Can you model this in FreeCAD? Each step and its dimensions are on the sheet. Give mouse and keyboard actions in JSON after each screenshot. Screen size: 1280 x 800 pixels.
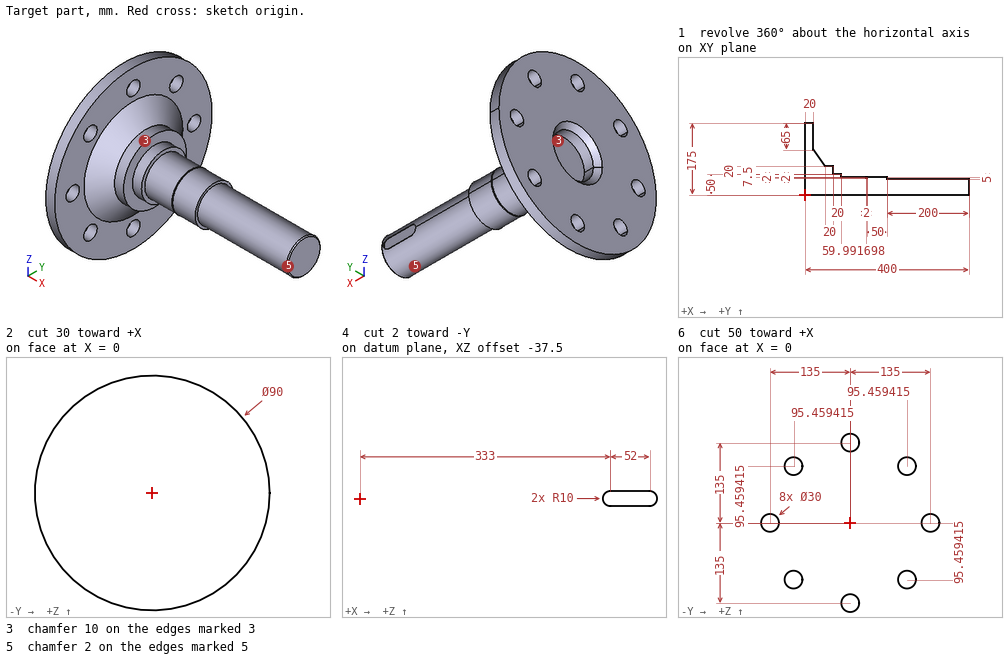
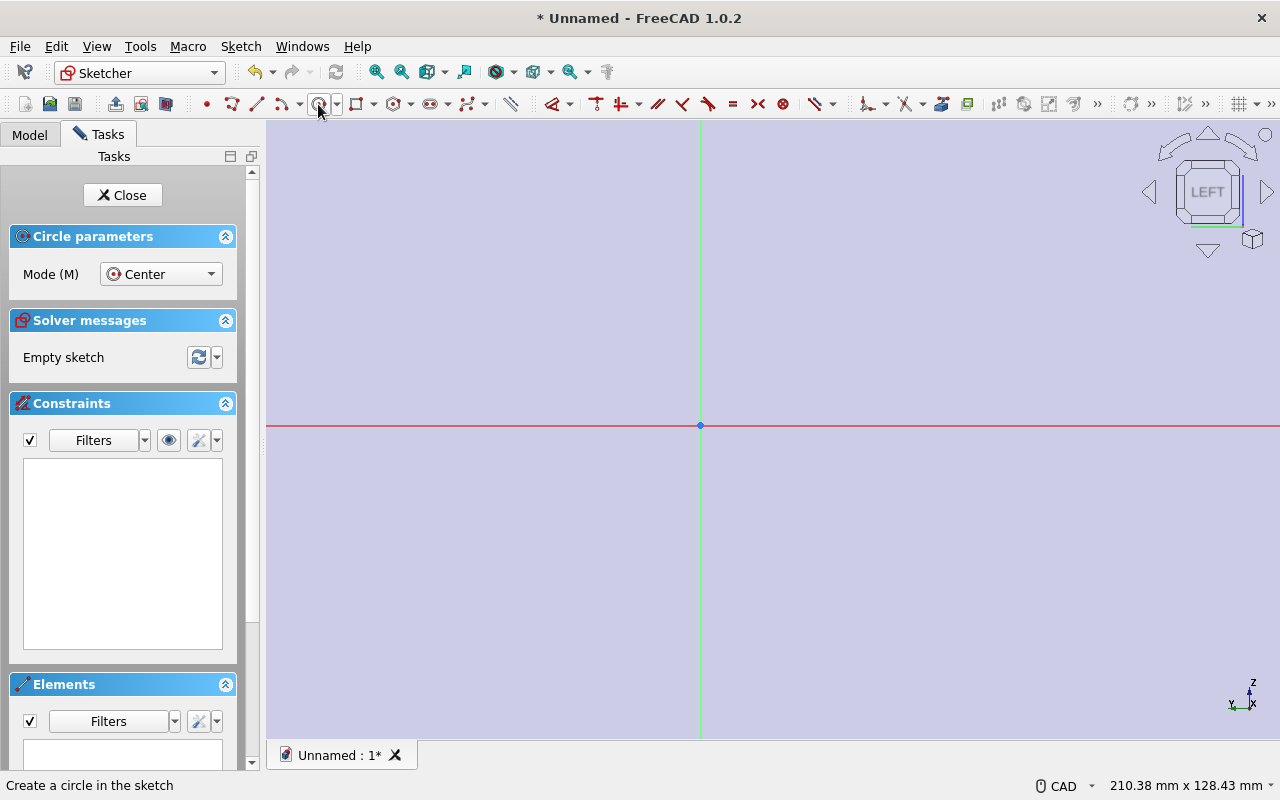
{"action": "left_click", "coordinate": [701, 426]}
{"action": "mouse_move", "coordinate": [854, 272]}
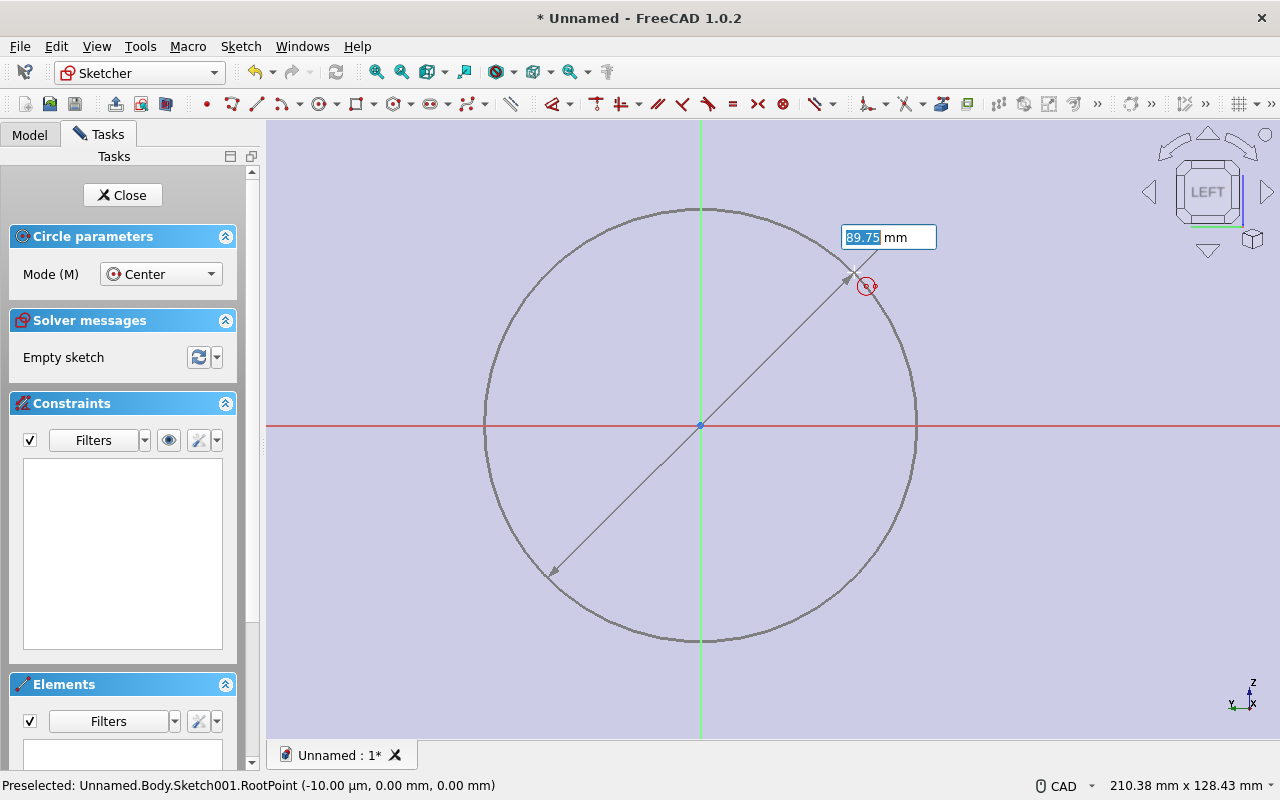
{"action": "type", "text": "90"}
{"action": "key", "text": "Return"}
{"action": "key", "text": "Escape"}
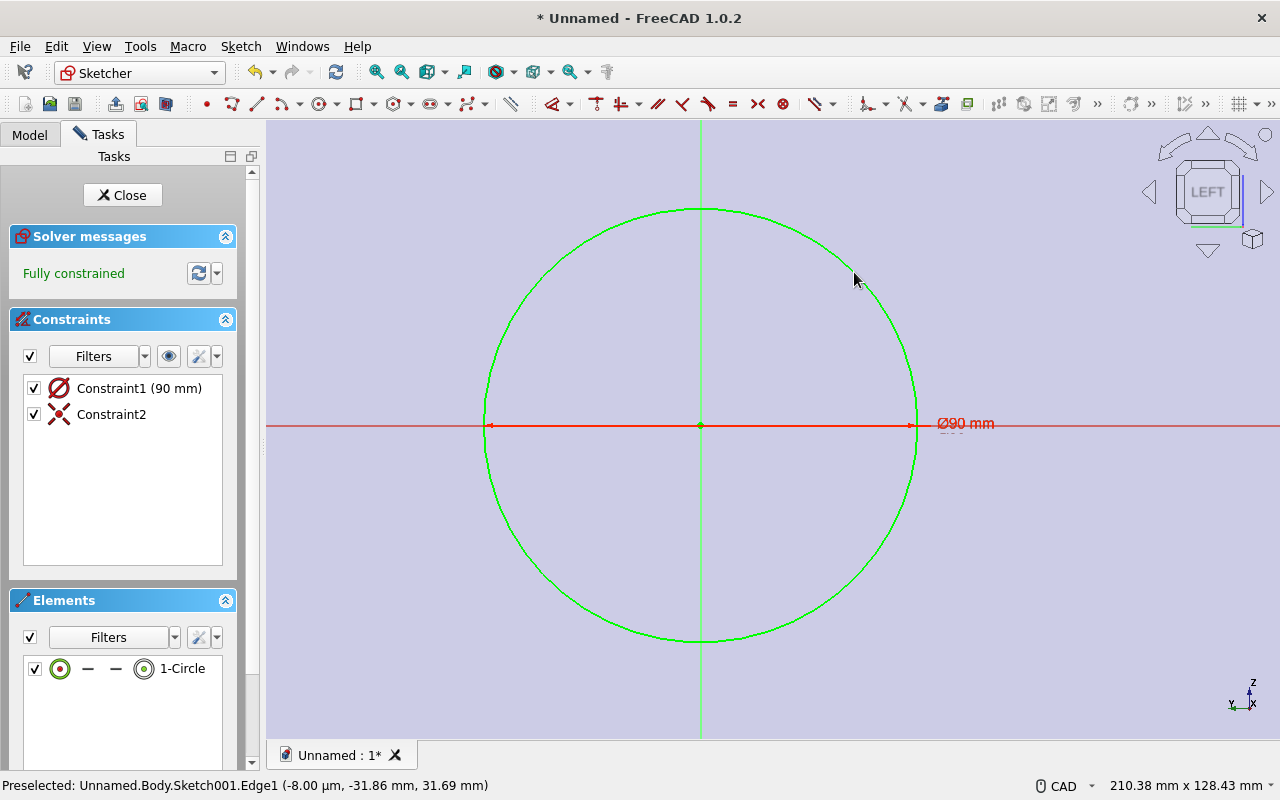
{"action": "left_click", "coordinate": [123, 195]}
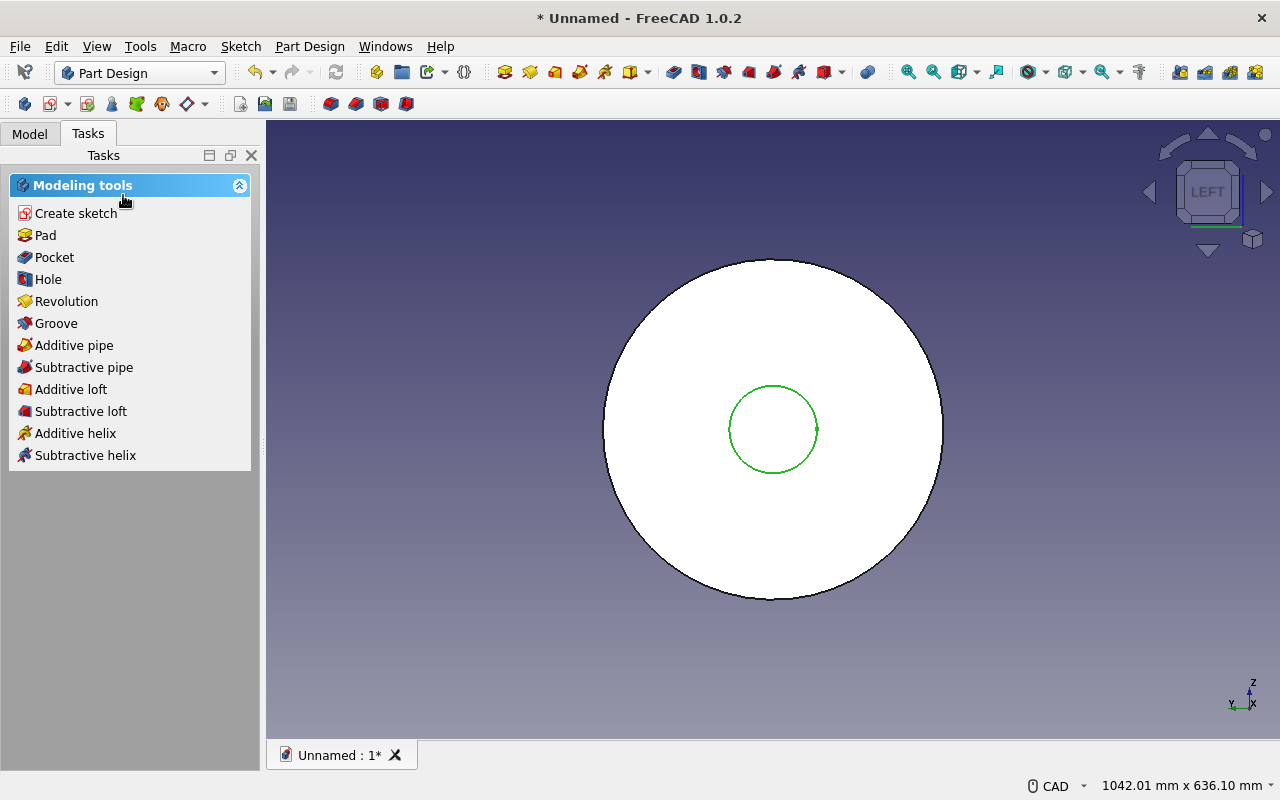
{"action": "left_click", "coordinate": [674, 72]}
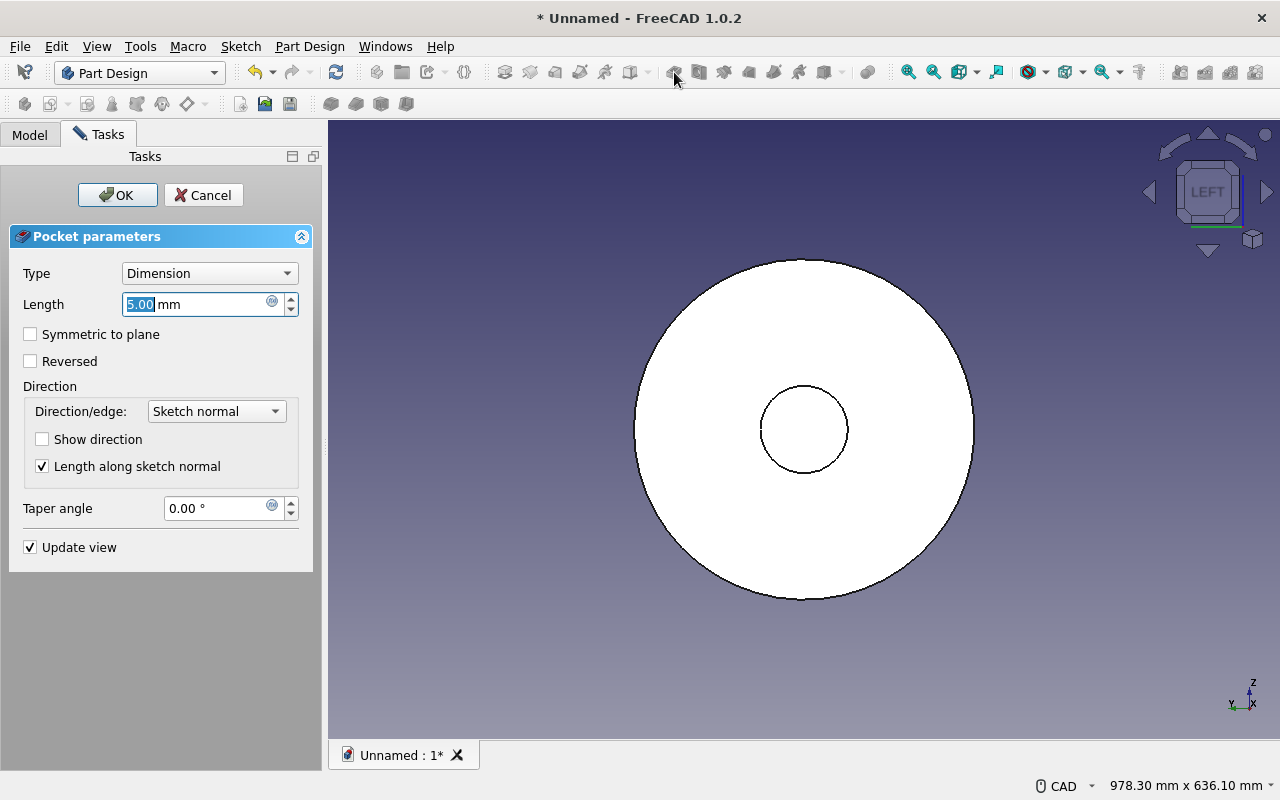
{"action": "type", "text": "30"}
{"action": "key", "text": "Tab"}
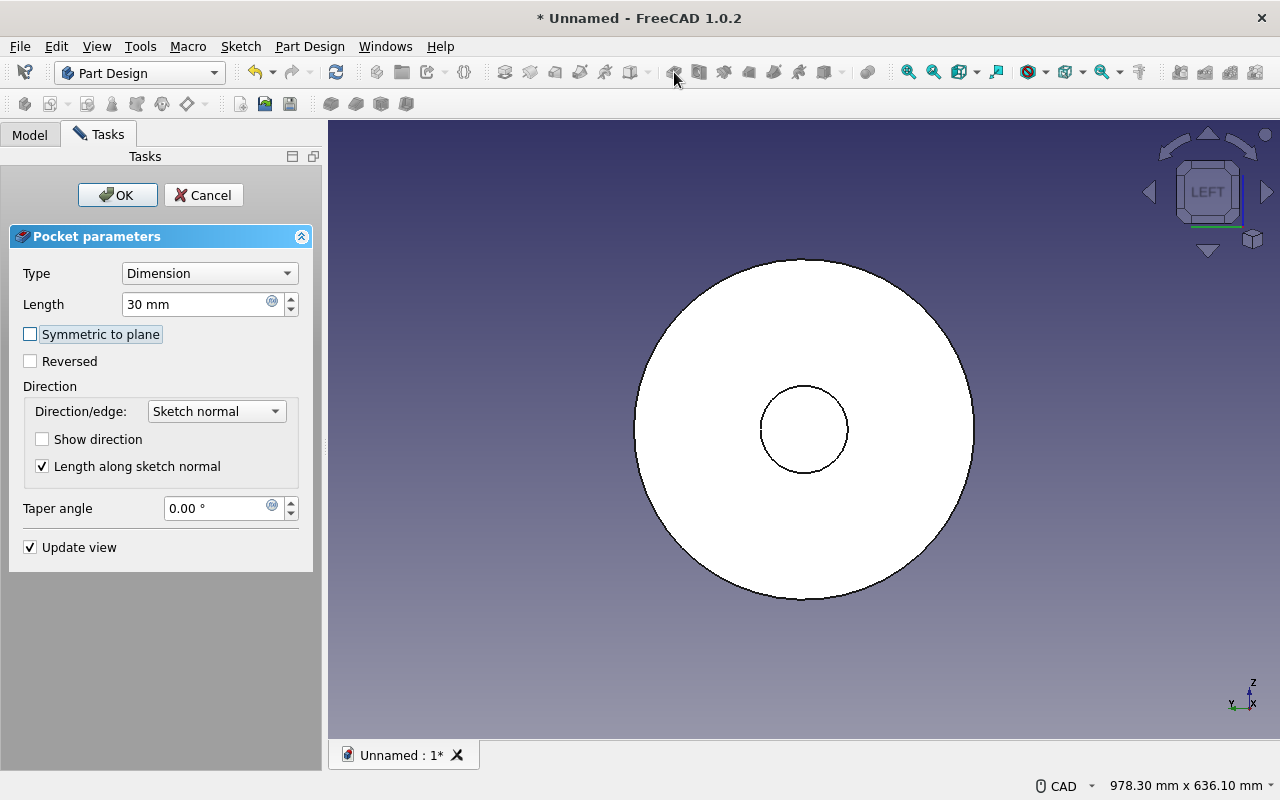
{"action": "left_click", "coordinate": [118, 195]}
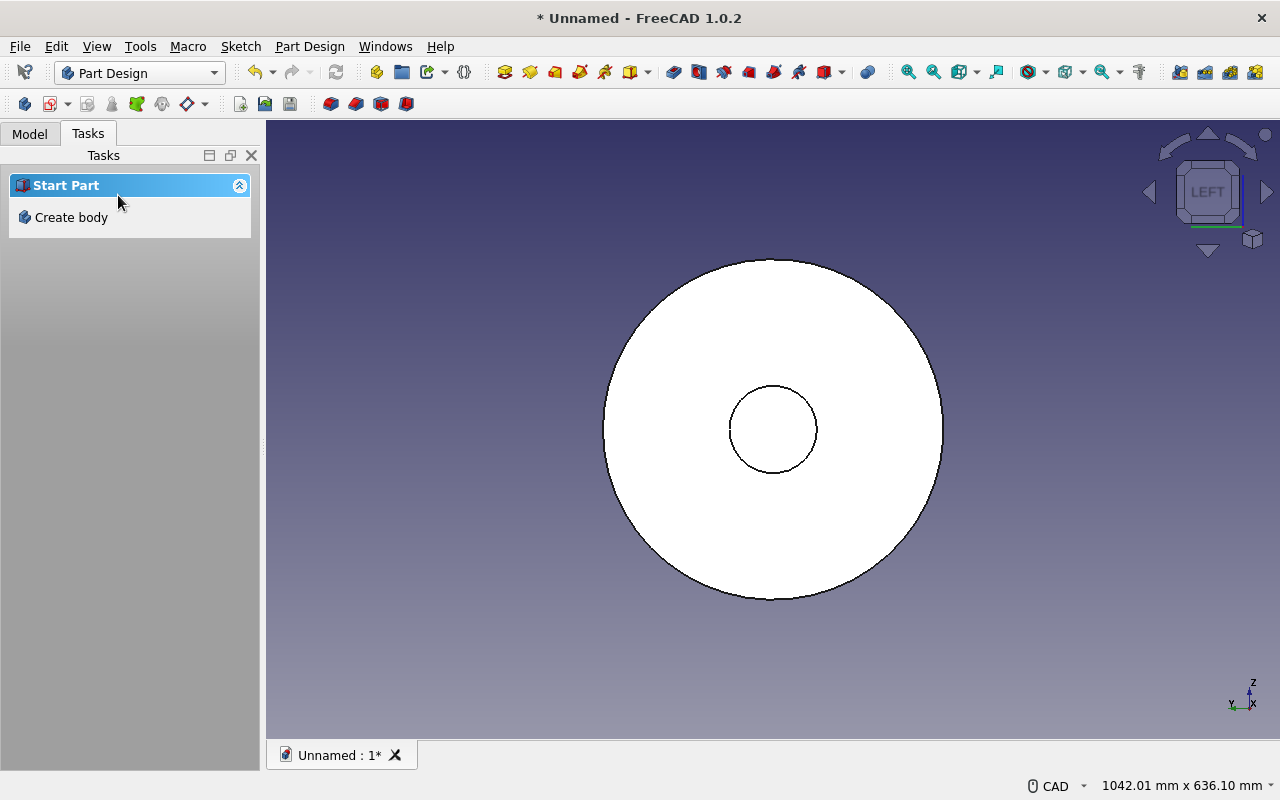
{"action": "left_click", "coordinate": [729, 428]}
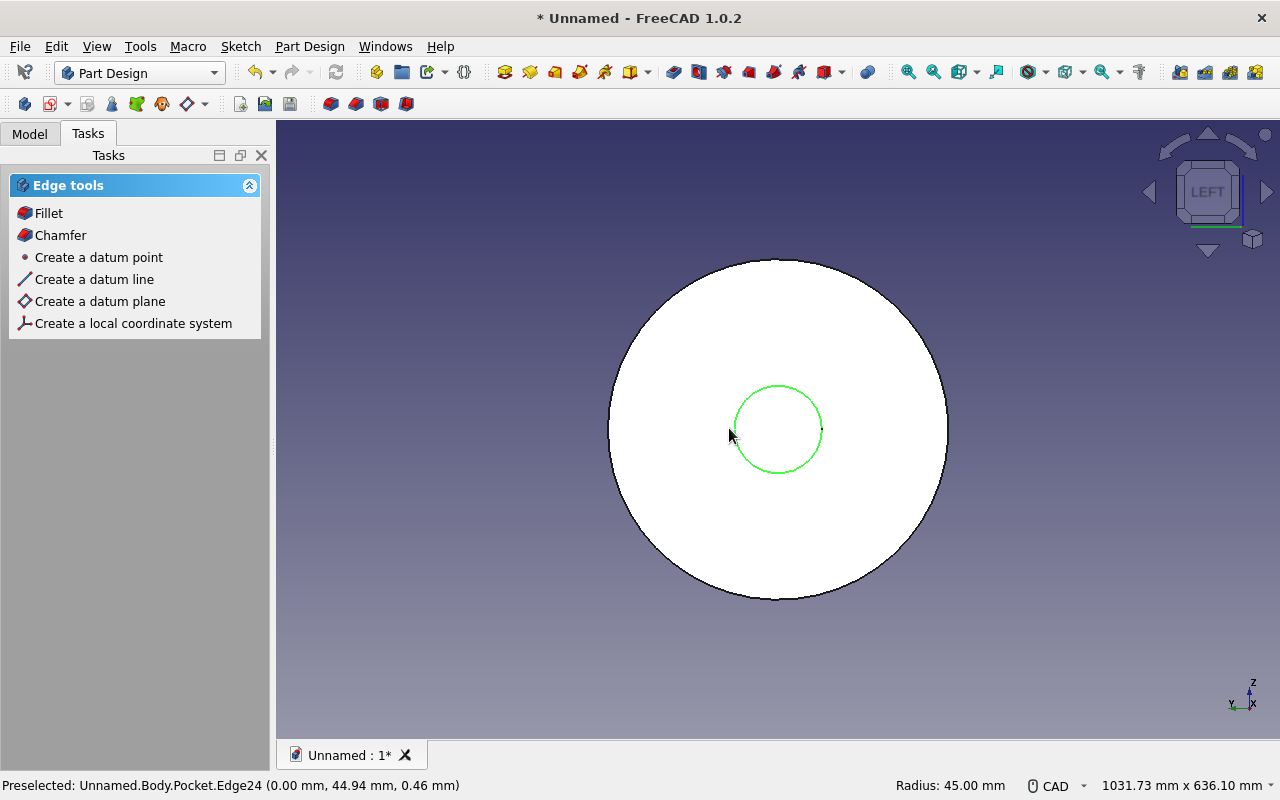
{"action": "left_click", "coordinate": [356, 104]}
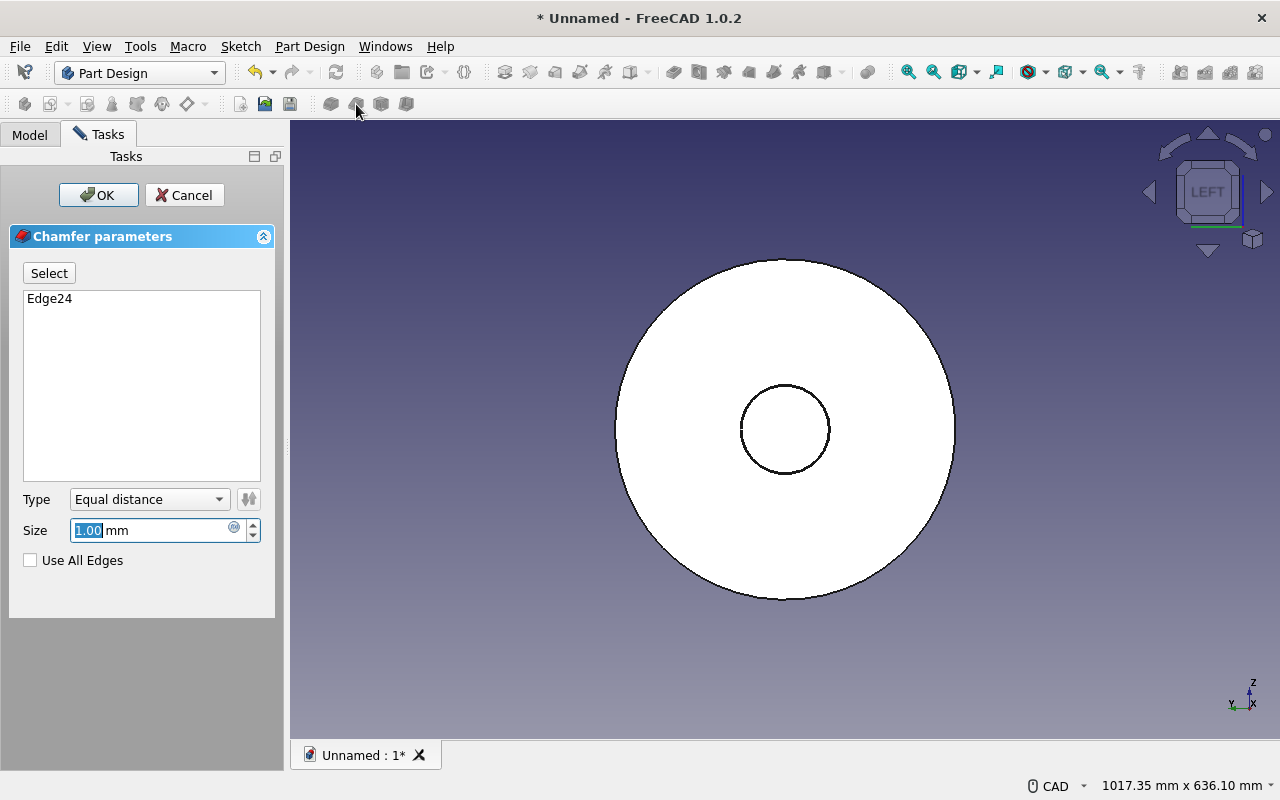
{"action": "type", "text": "10"}
{"action": "key", "text": "Tab"}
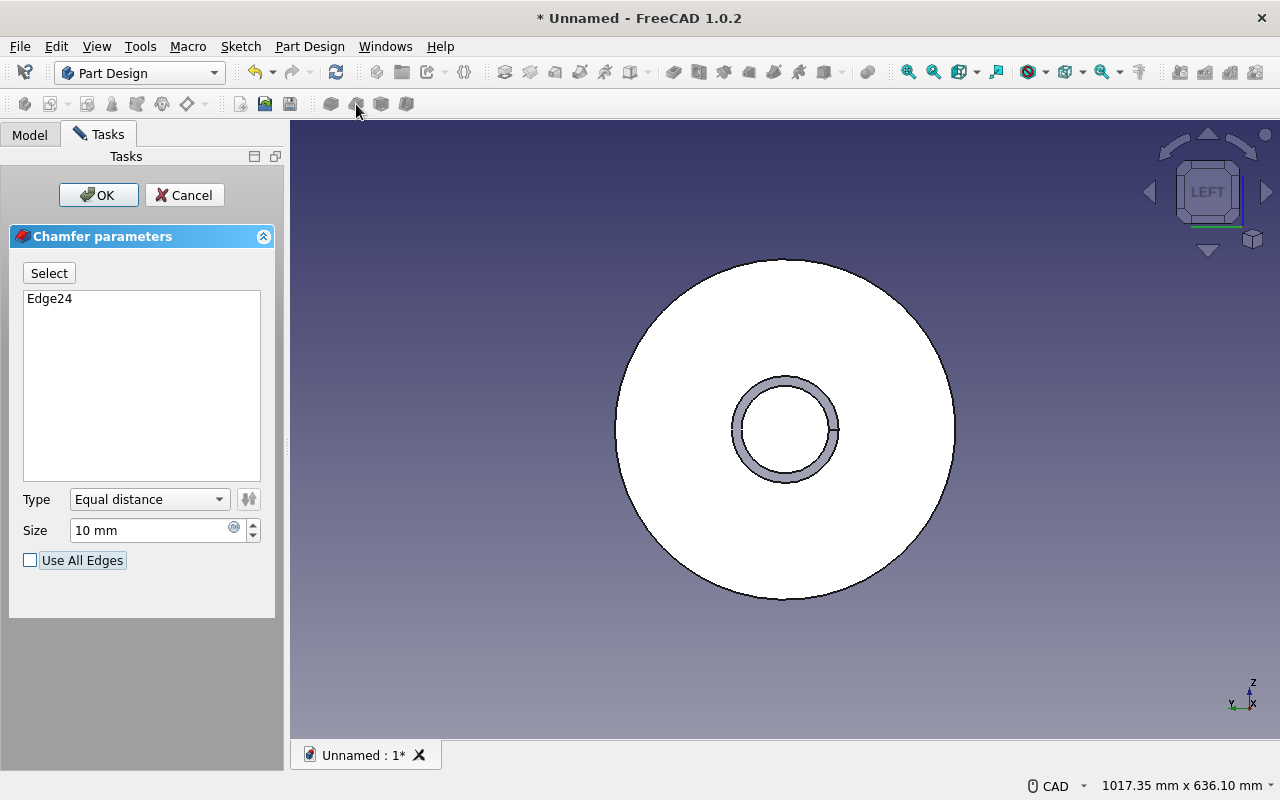
{"action": "left_click", "coordinate": [99, 195]}